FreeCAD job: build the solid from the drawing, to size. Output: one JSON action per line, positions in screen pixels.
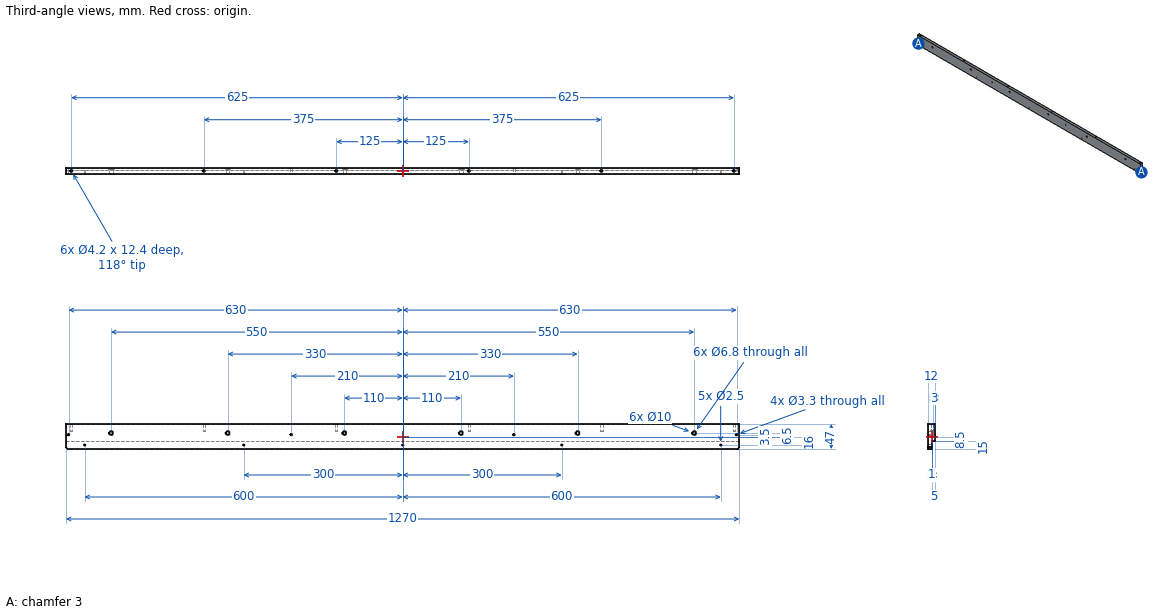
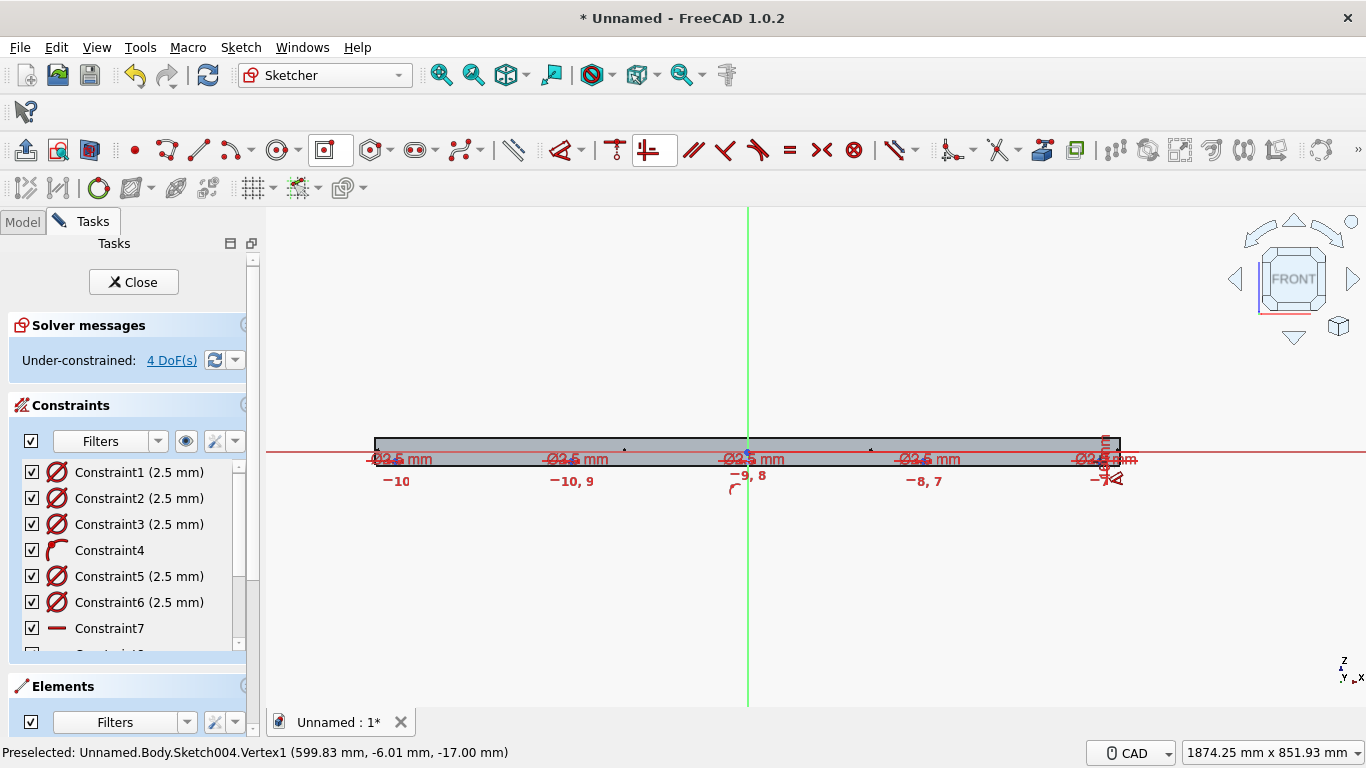
{"action": "left_click", "coordinate": [1100, 461]}
{"action": "left_click", "coordinate": [924, 418]}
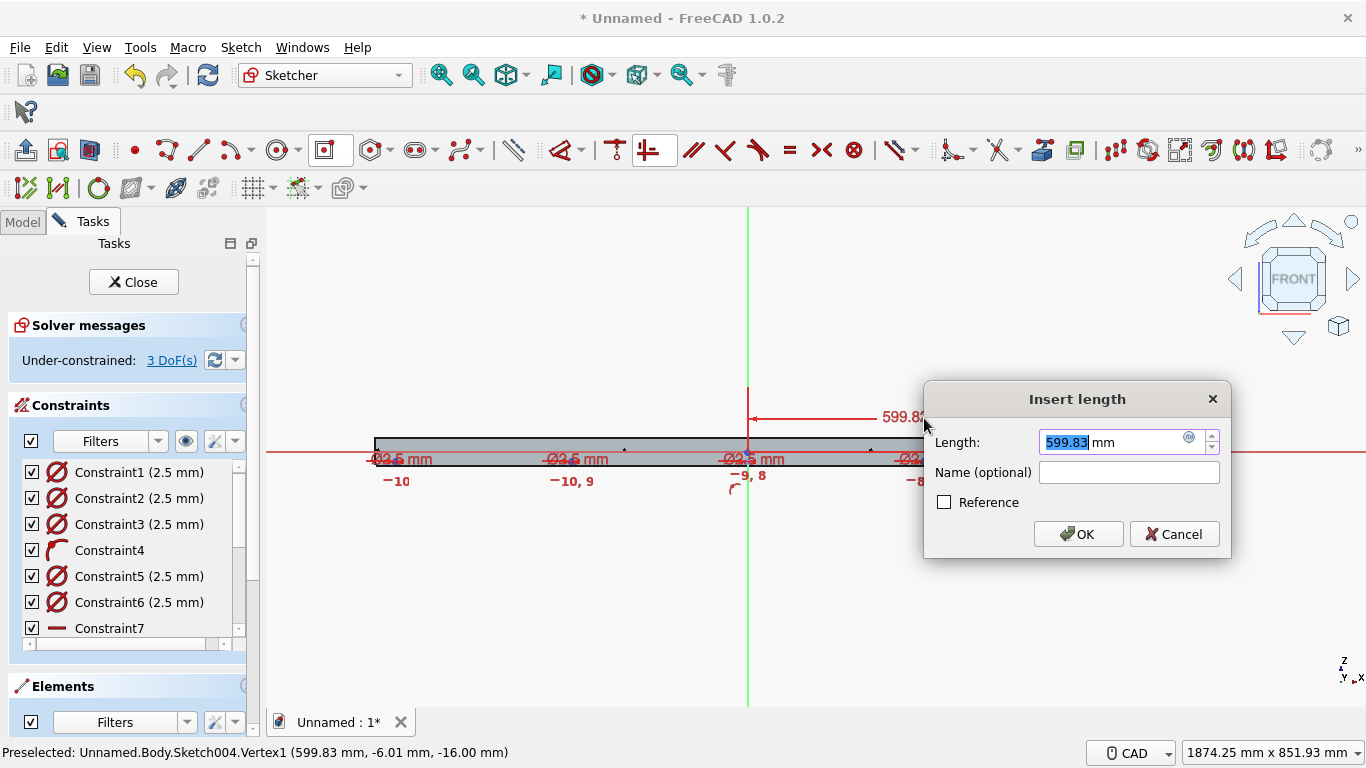
{"action": "type", "text": "600"}
{"action": "key", "text": "Return"}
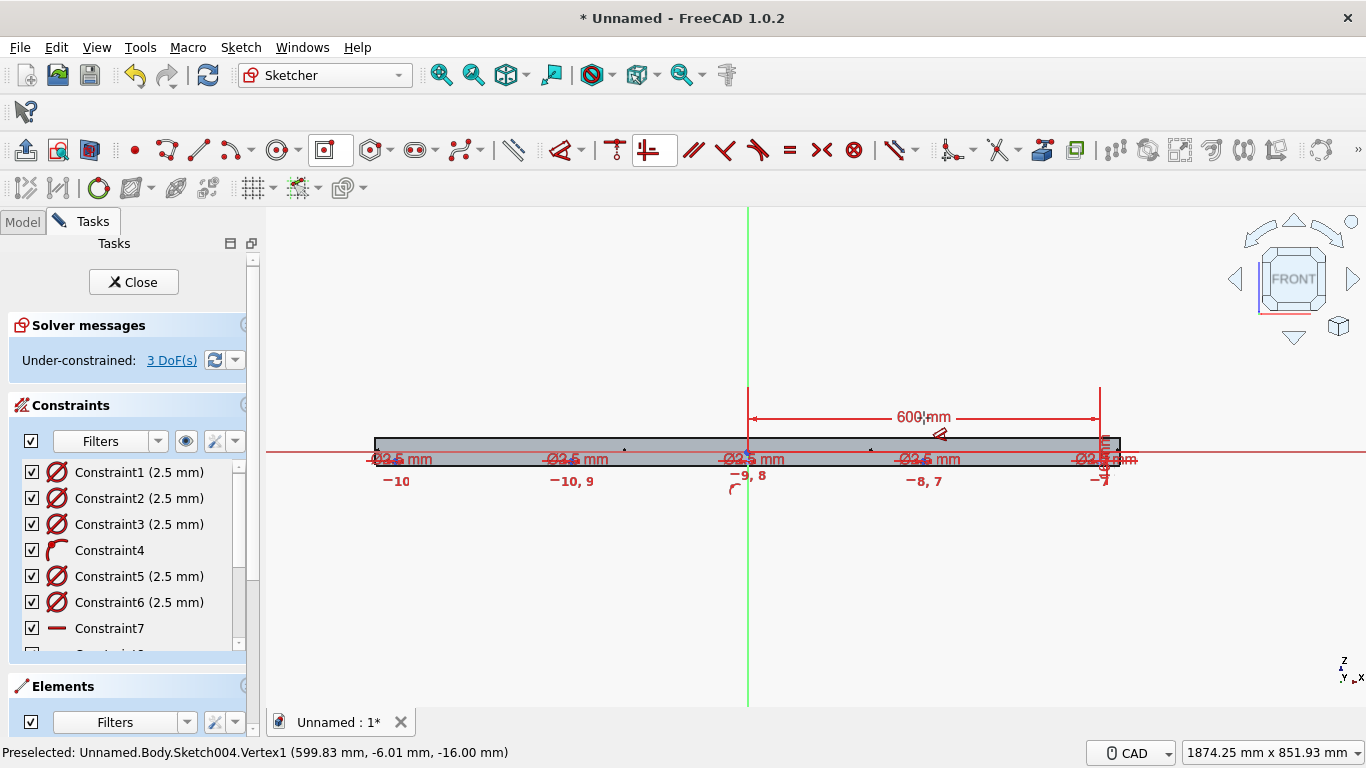
{"action": "left_click", "coordinate": [924, 461]}
{"action": "left_click", "coordinate": [836, 418]}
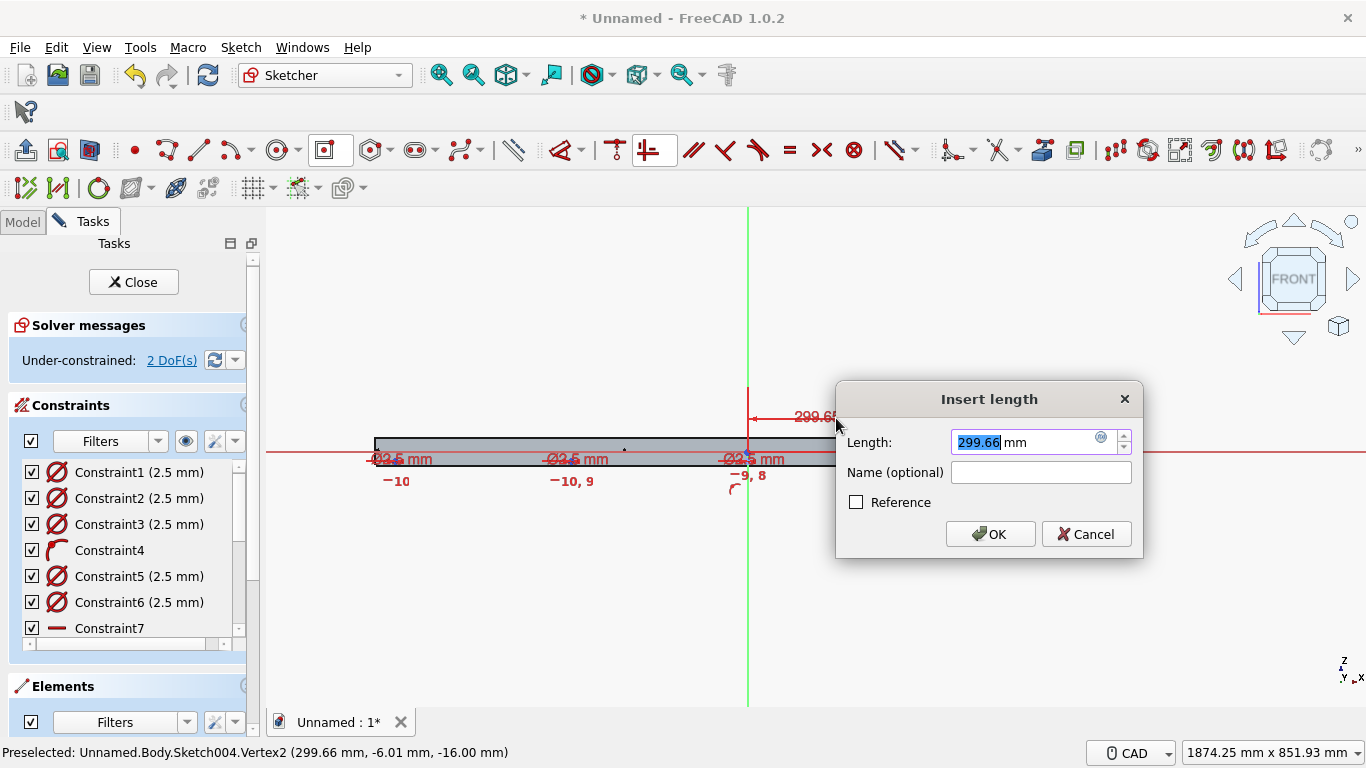
{"action": "type", "text": "300"}
{"action": "key", "text": "Return"}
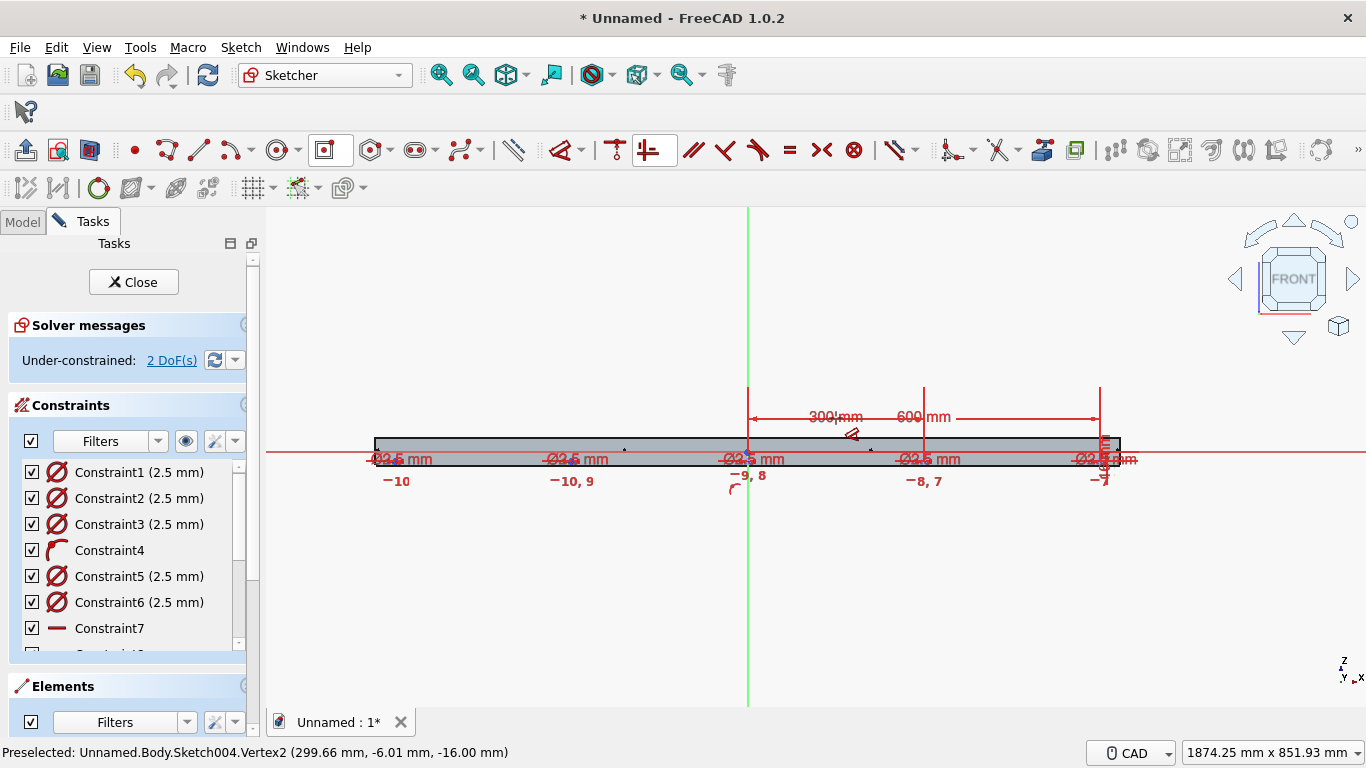
{"action": "left_click", "coordinate": [571, 461]}
{"action": "left_click", "coordinate": [660, 418]}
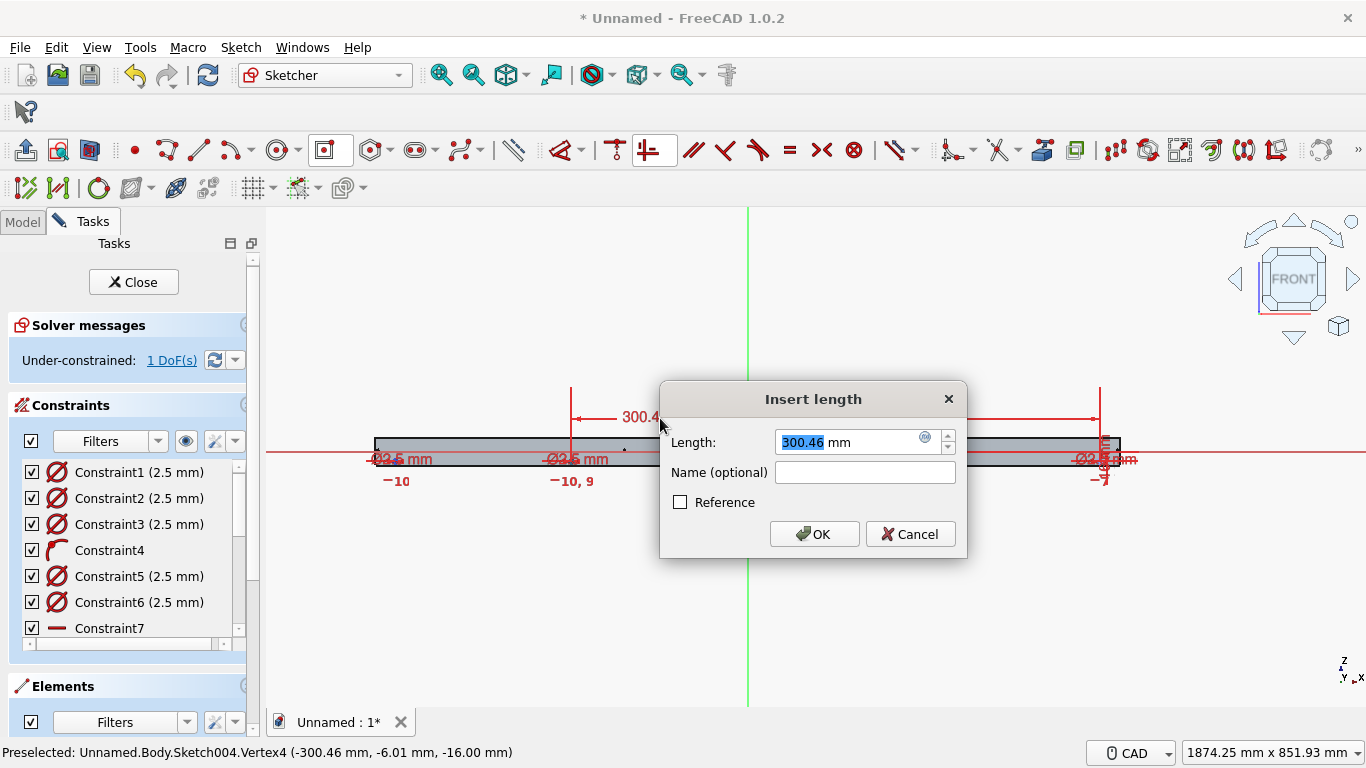
{"action": "type", "text": "300"}
{"action": "key", "text": "Return"}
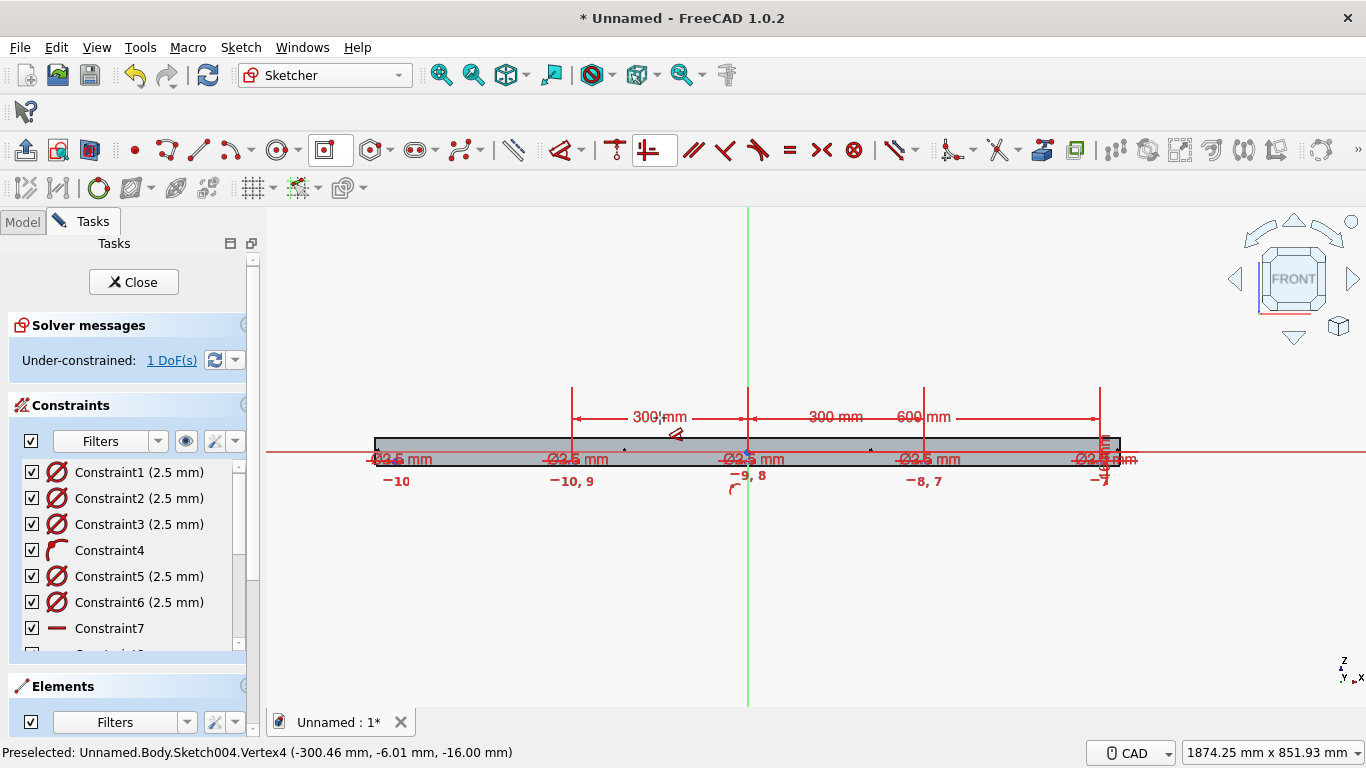
{"action": "left_click", "coordinate": [395, 461]}
{"action": "left_click", "coordinate": [572, 418]}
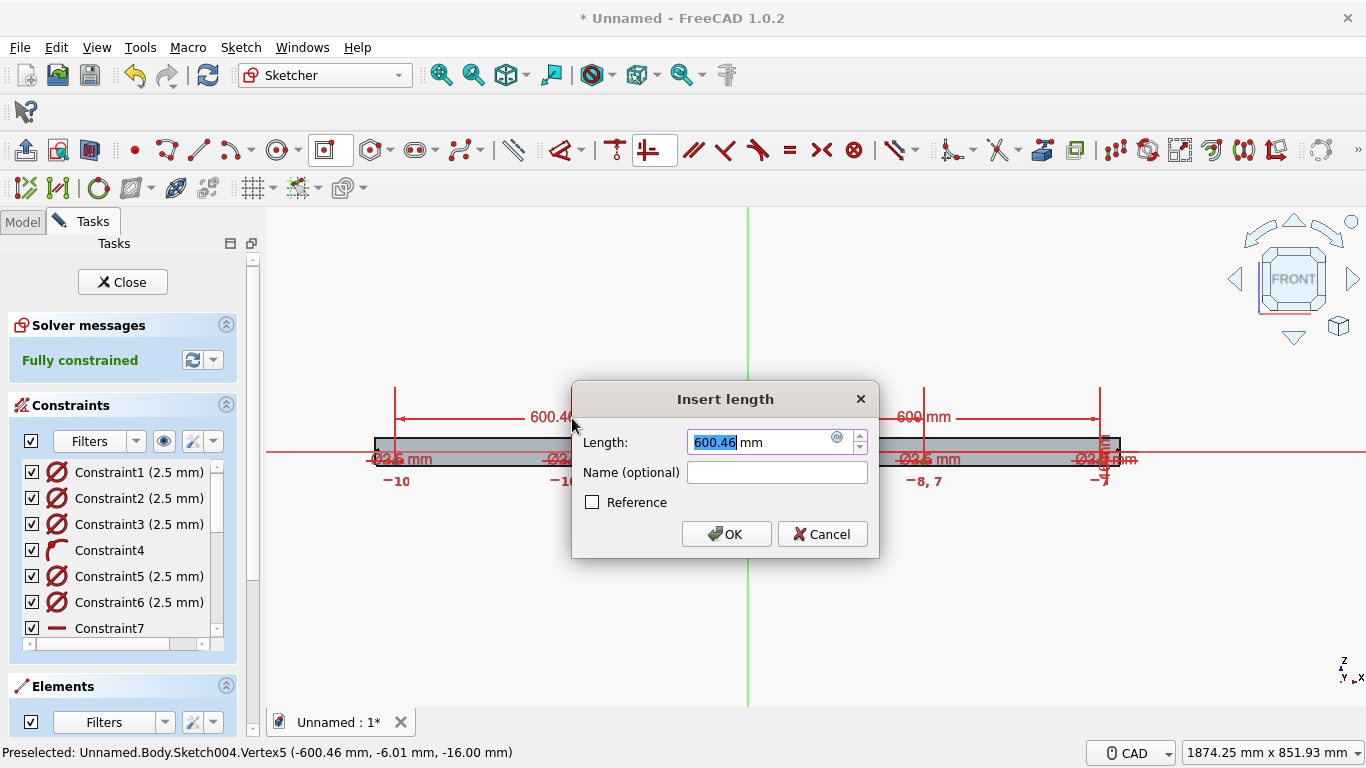
{"action": "type", "text": "600"}
{"action": "key", "text": "Return"}
{"action": "key", "text": "Escape"}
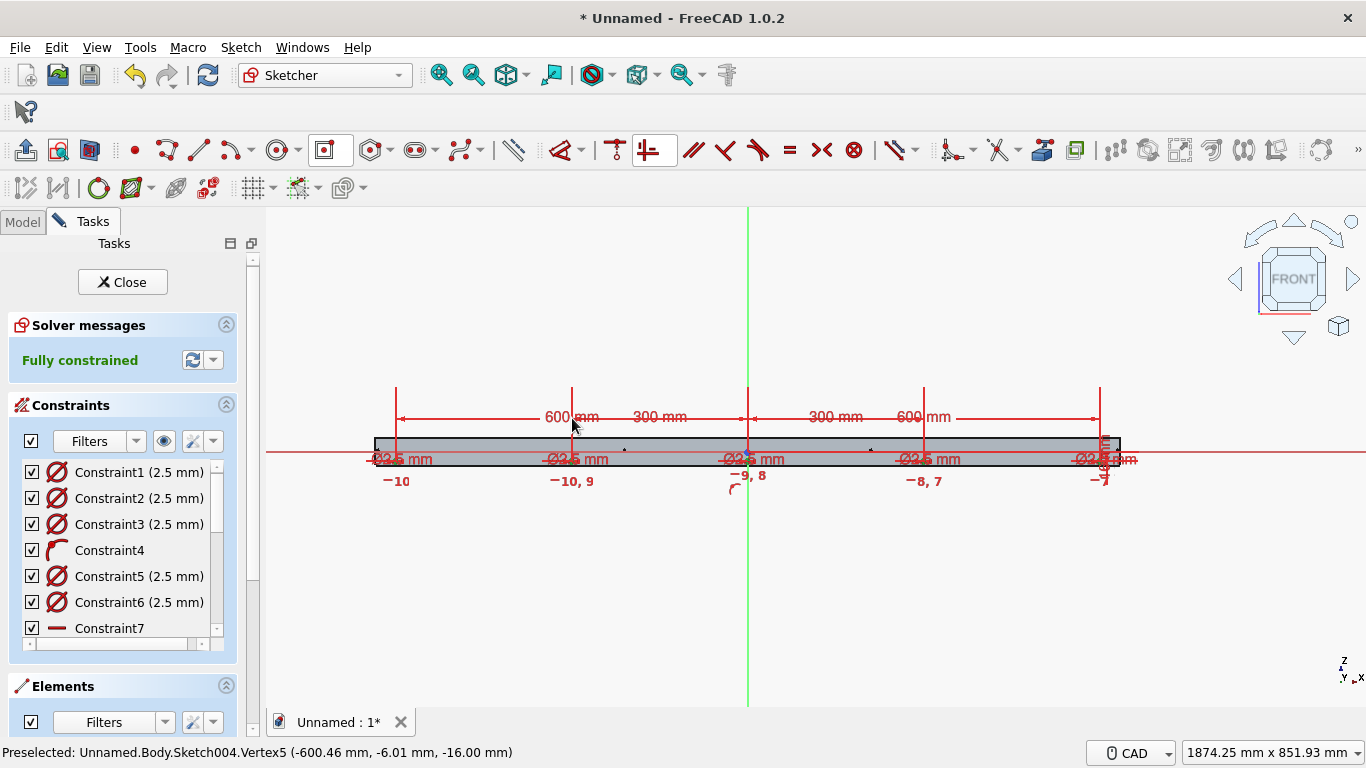
{"action": "left_click", "coordinate": [123, 282]}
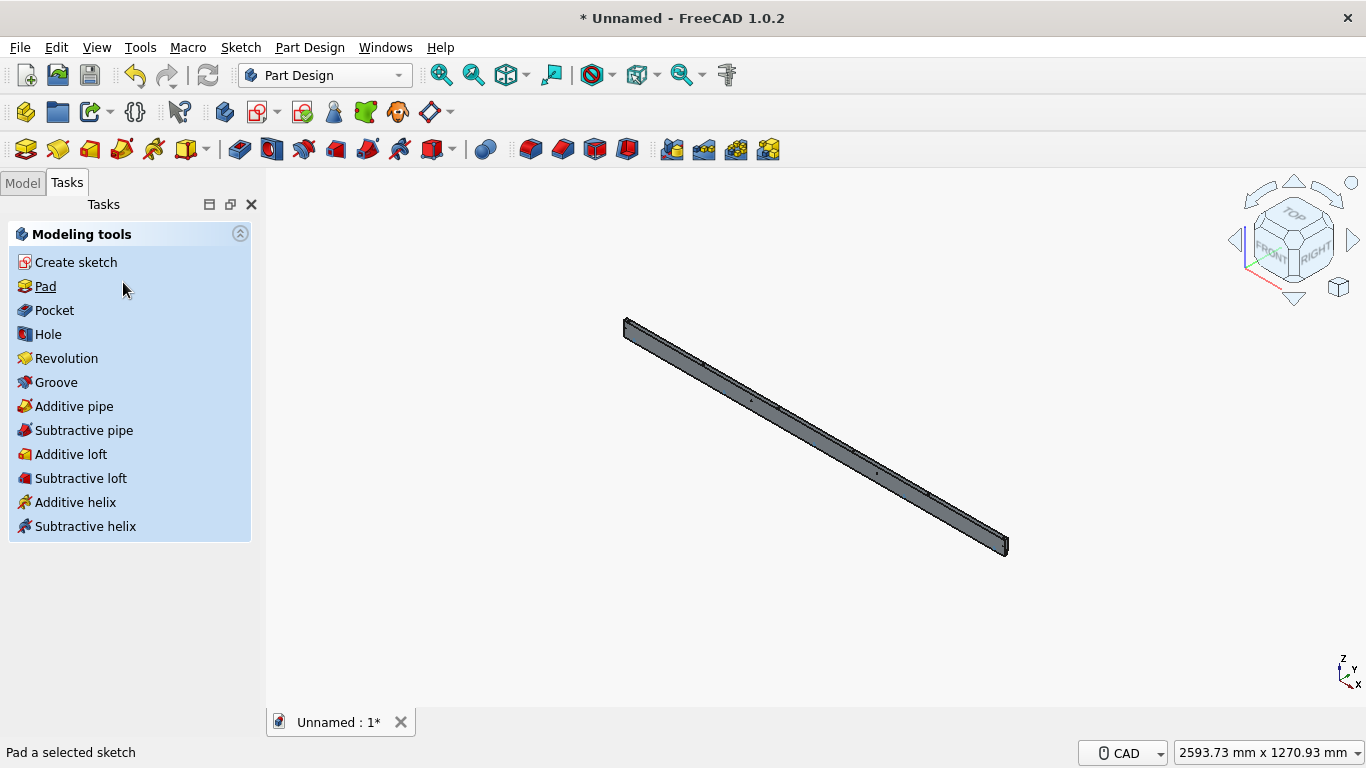
{"action": "left_click", "coordinate": [240, 150]}